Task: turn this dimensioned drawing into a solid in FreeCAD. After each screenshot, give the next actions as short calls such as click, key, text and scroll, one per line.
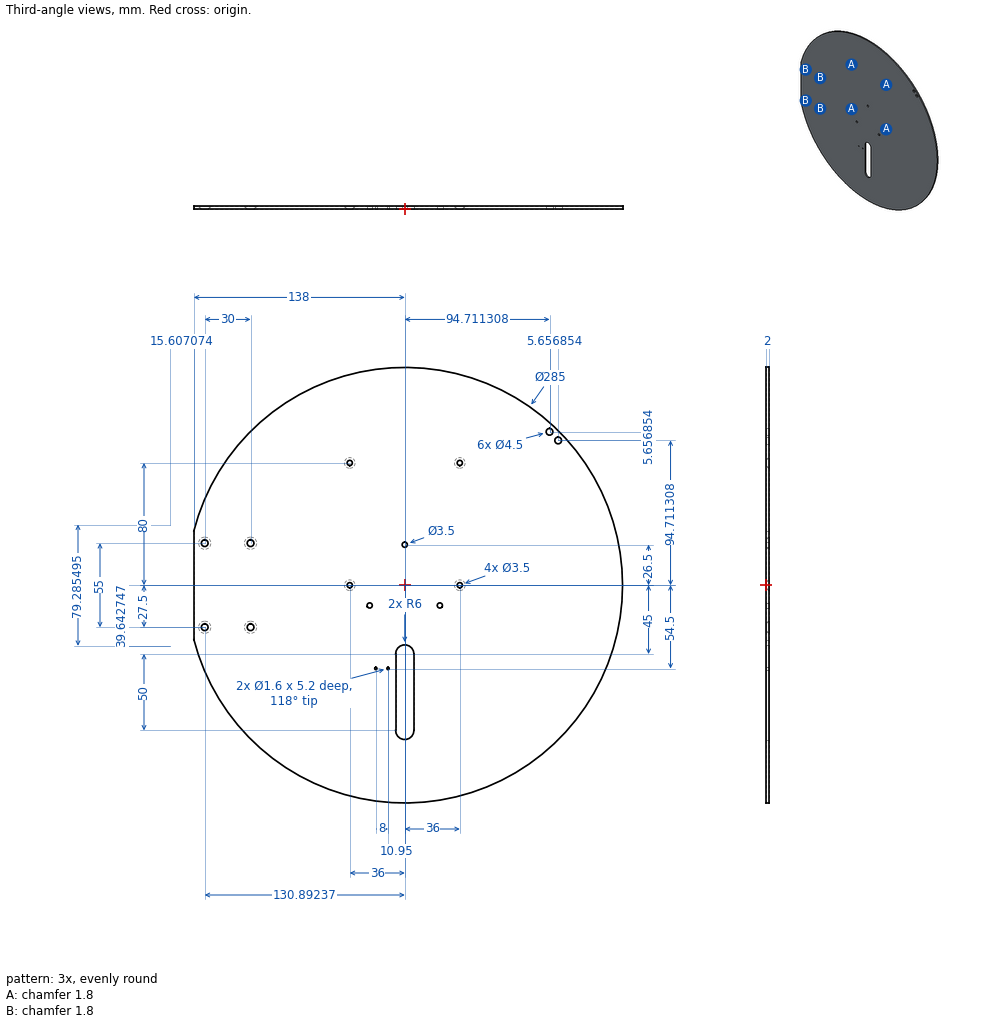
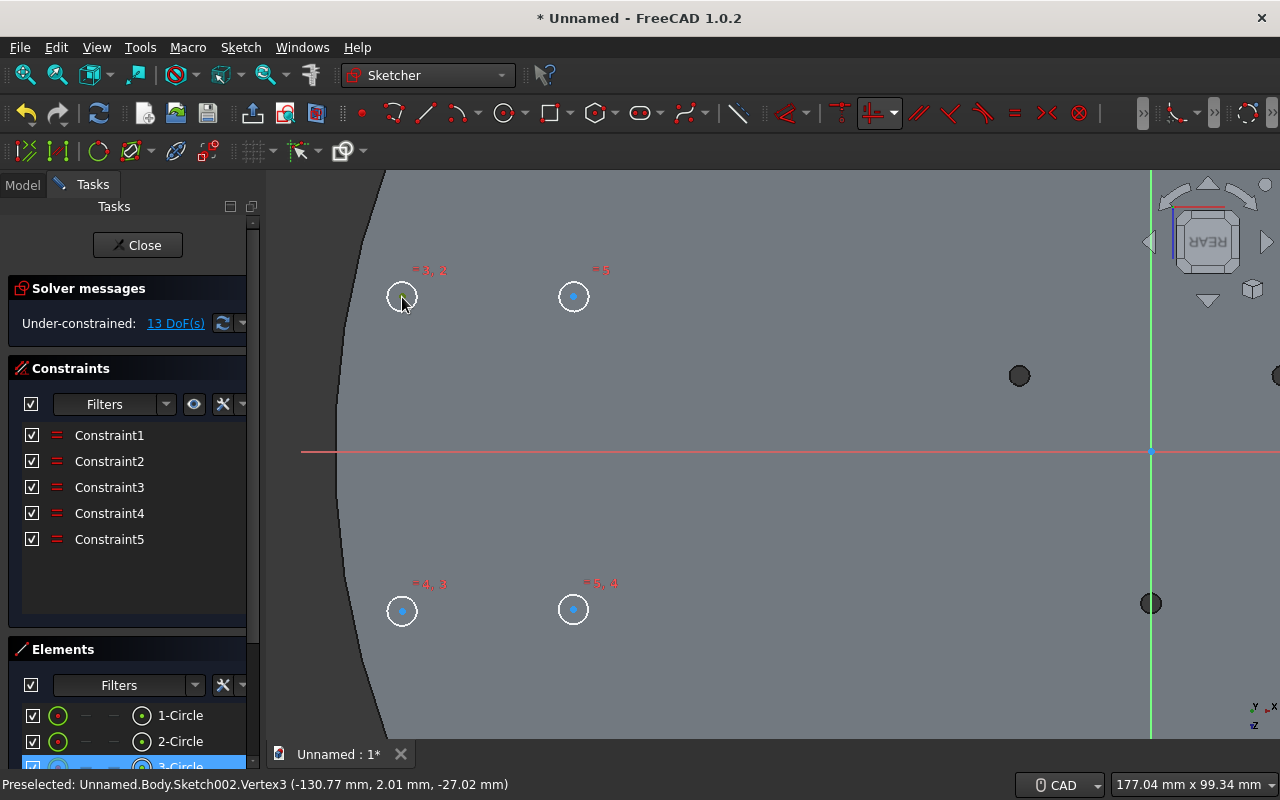
click(402, 611)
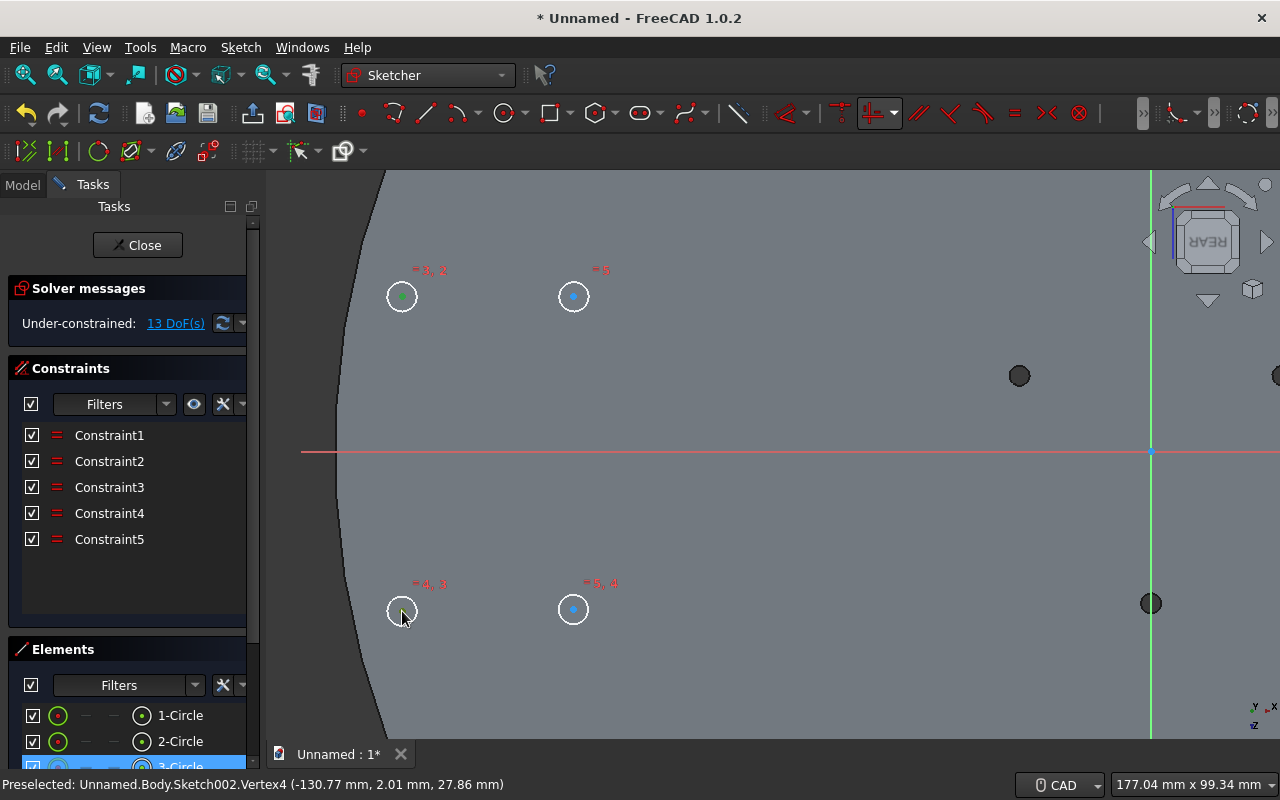
click(896, 114)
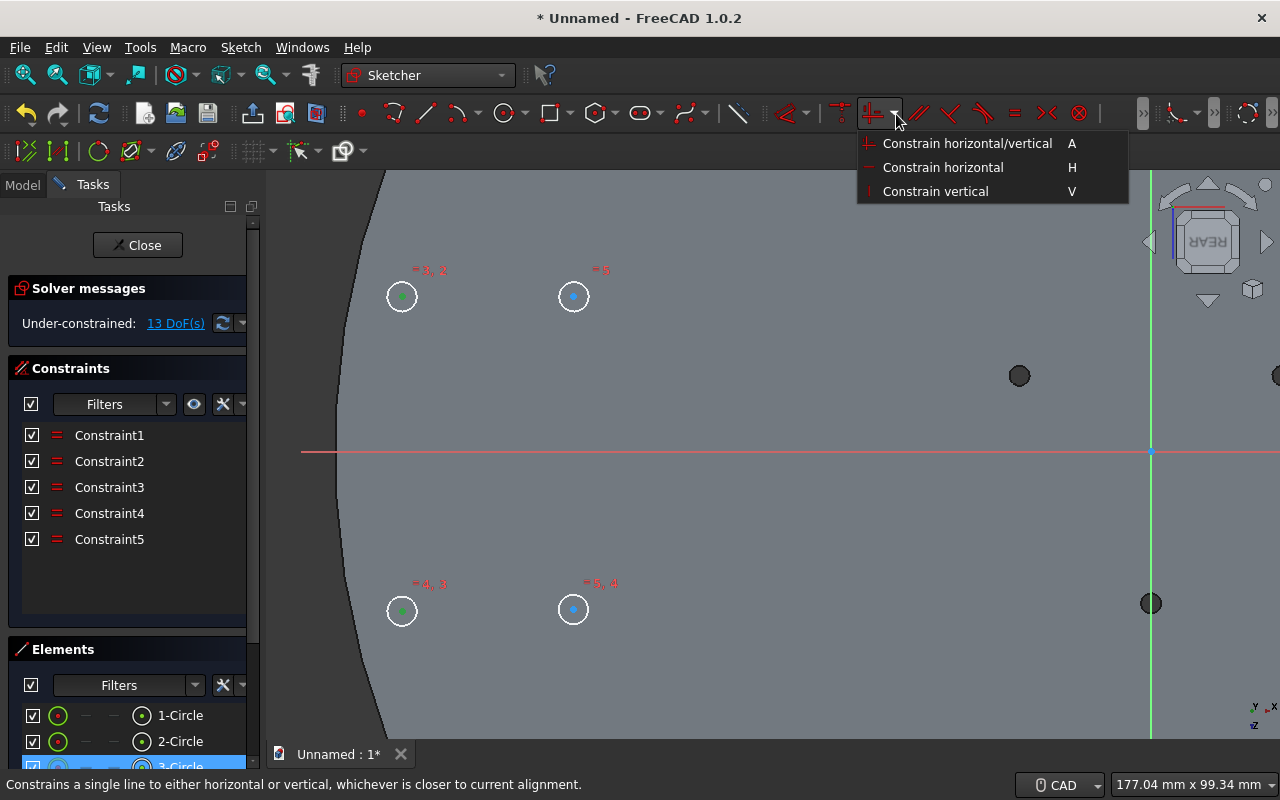
click(993, 191)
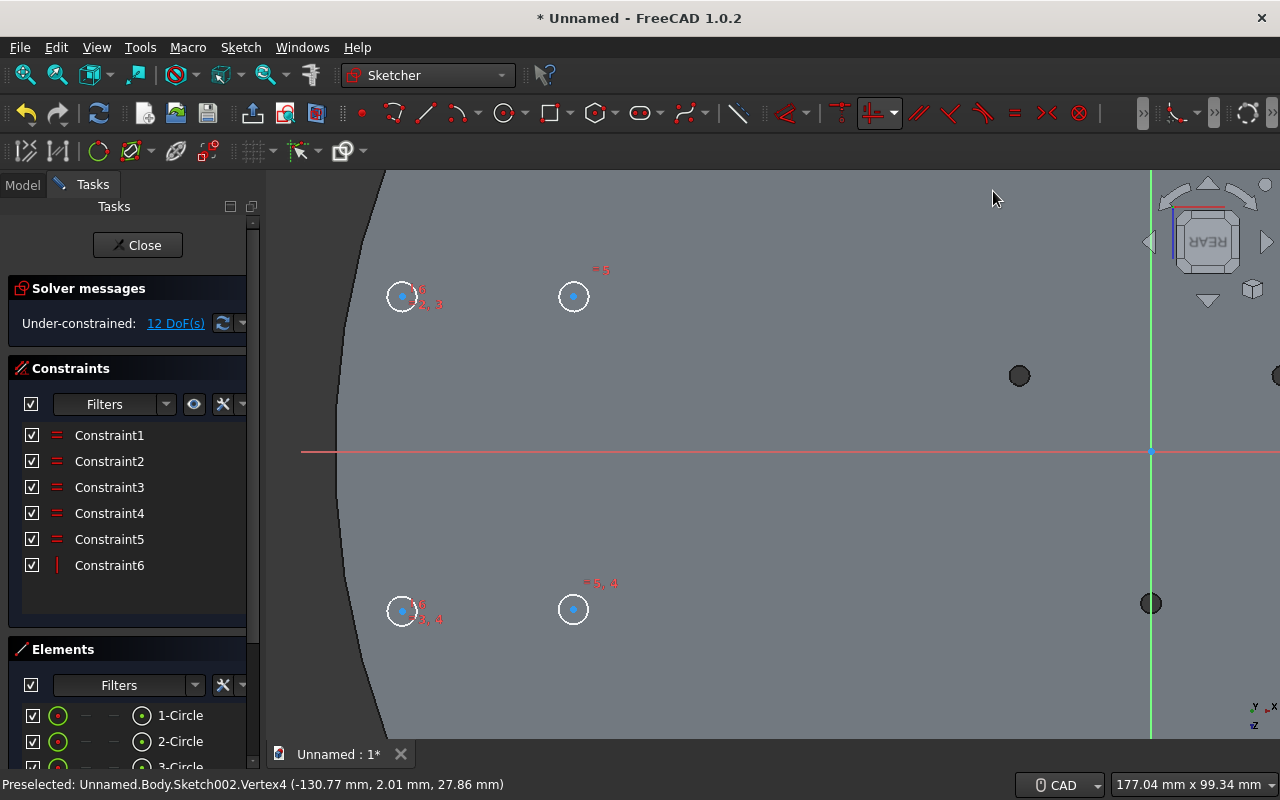
click(402, 611)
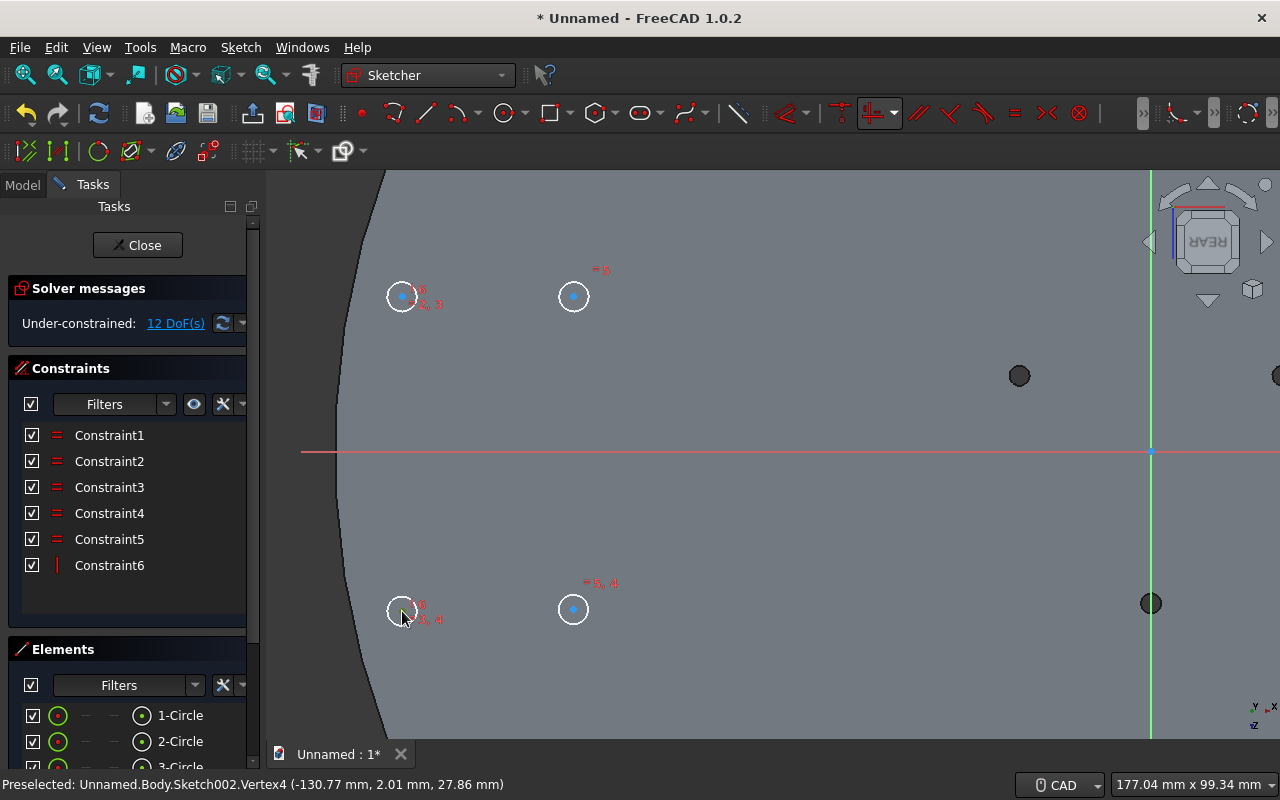
click(573, 610)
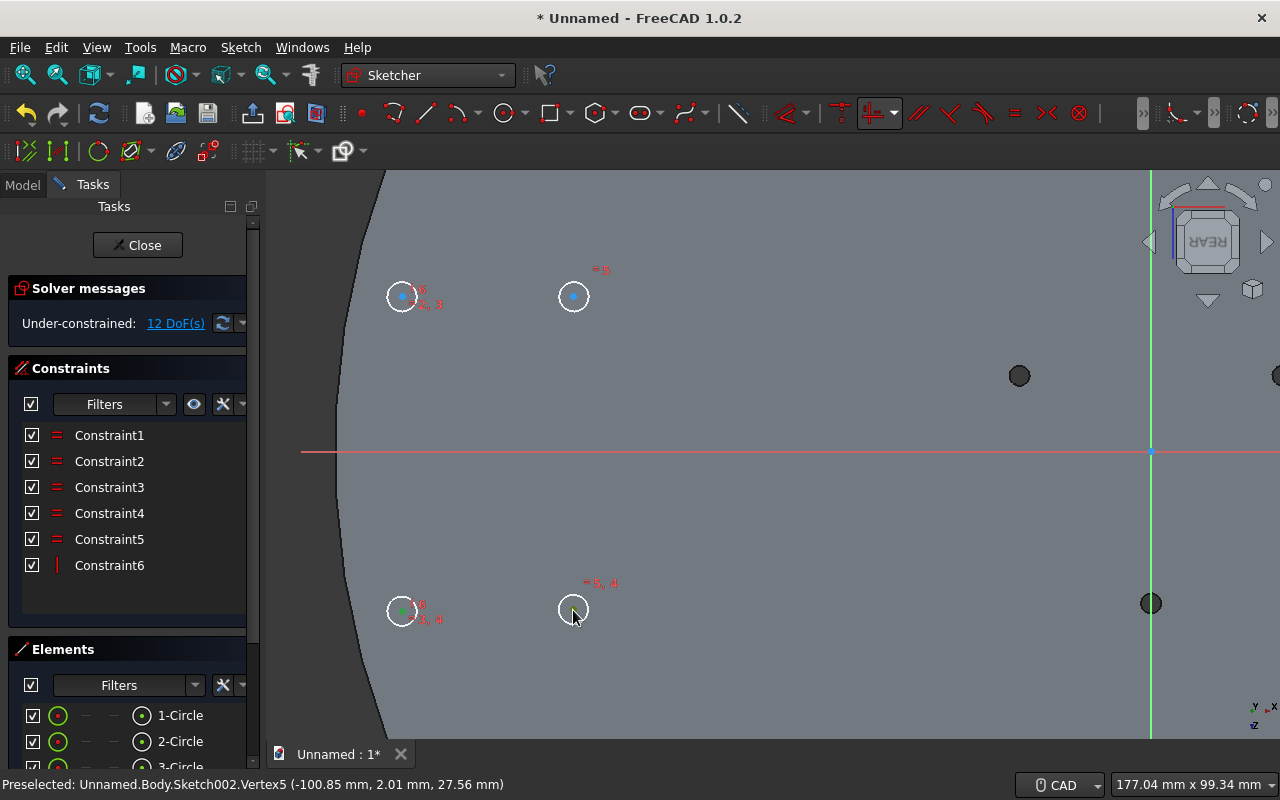
click(896, 114)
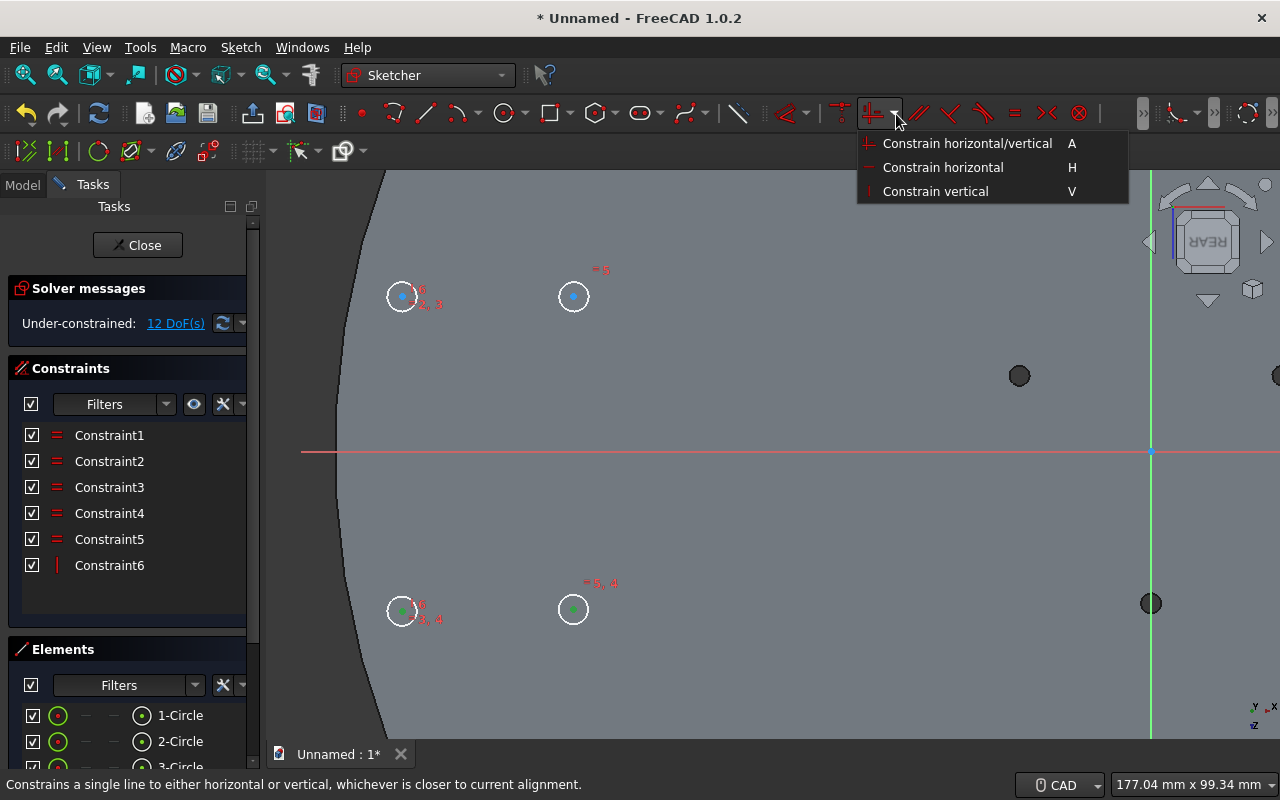
click(993, 167)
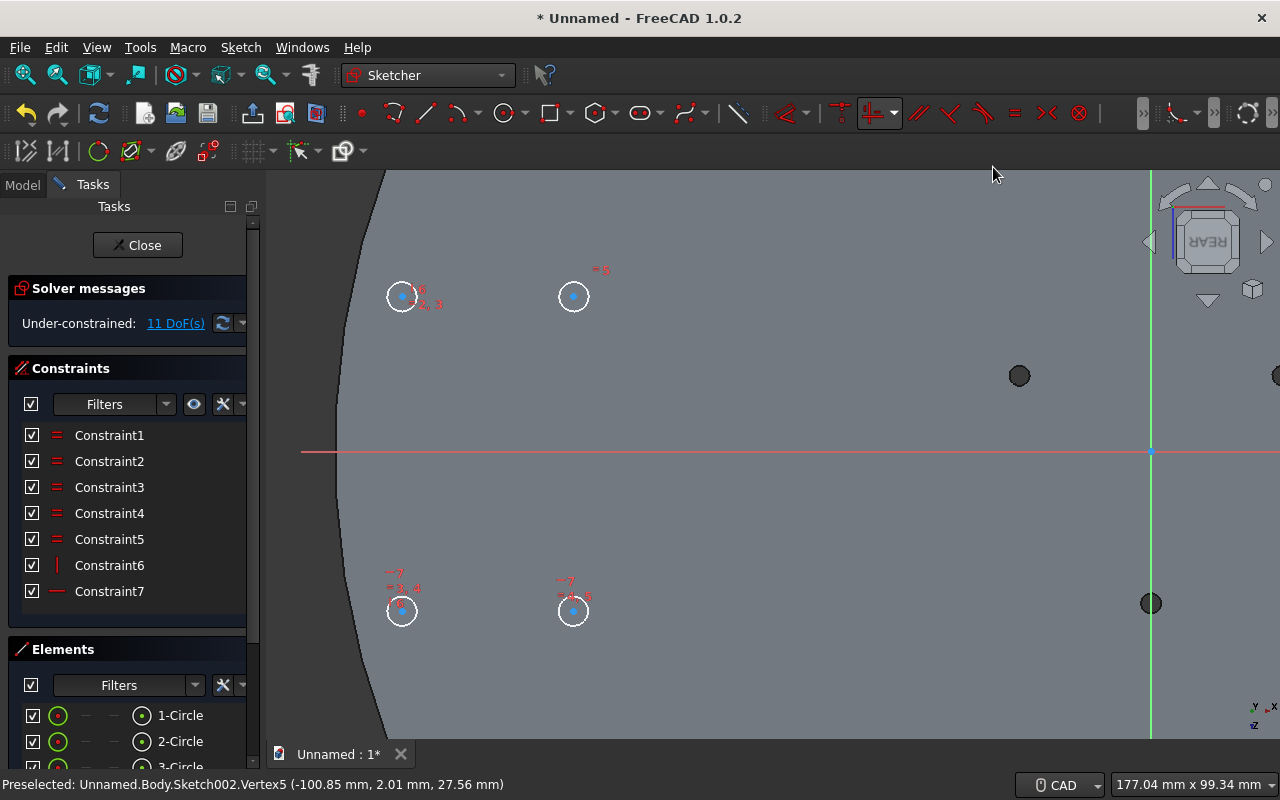
click(573, 611)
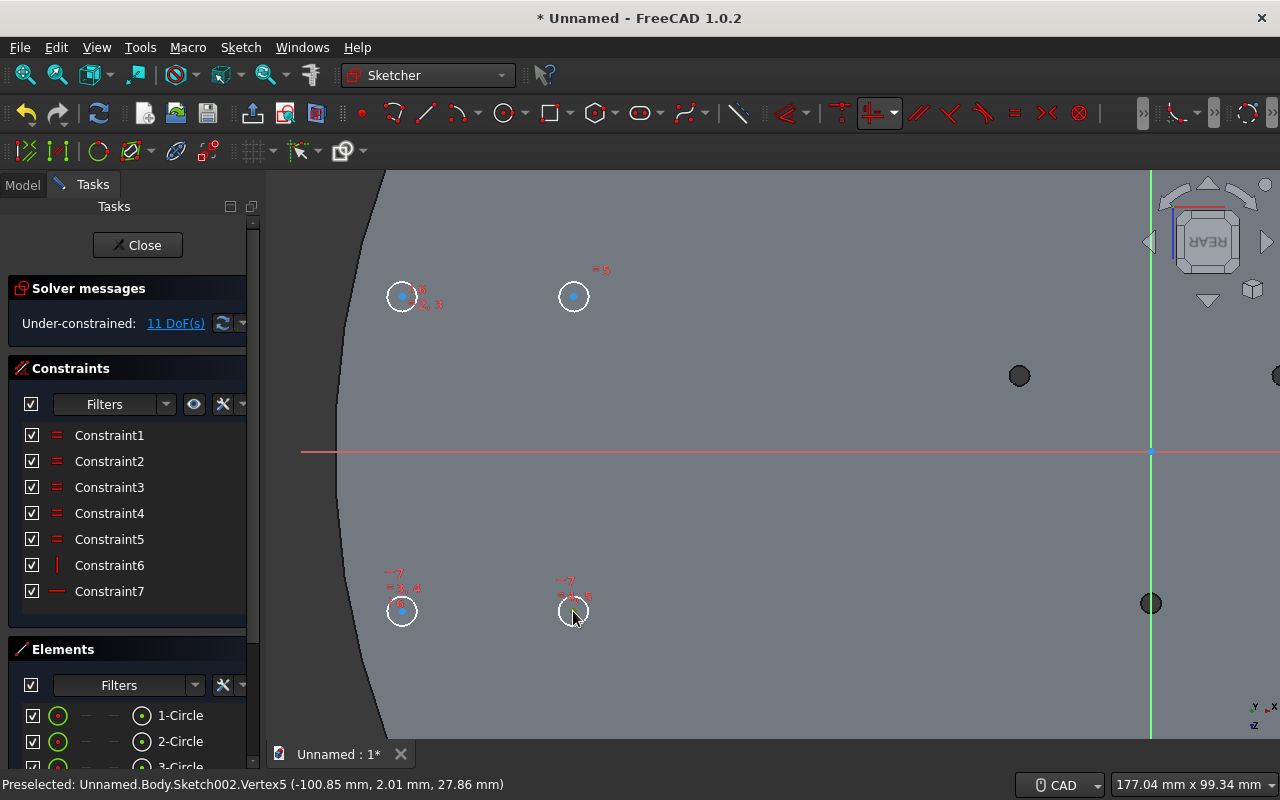
click(574, 297)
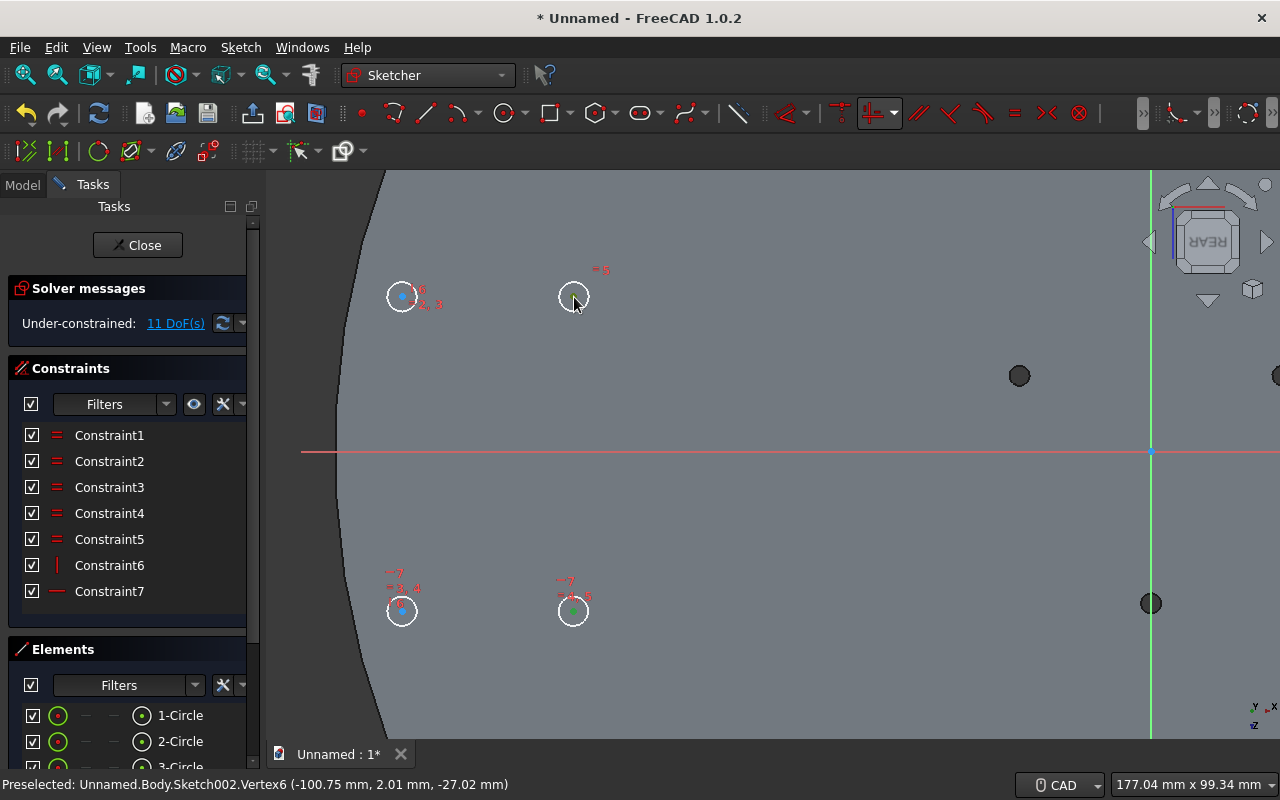
click(896, 114)